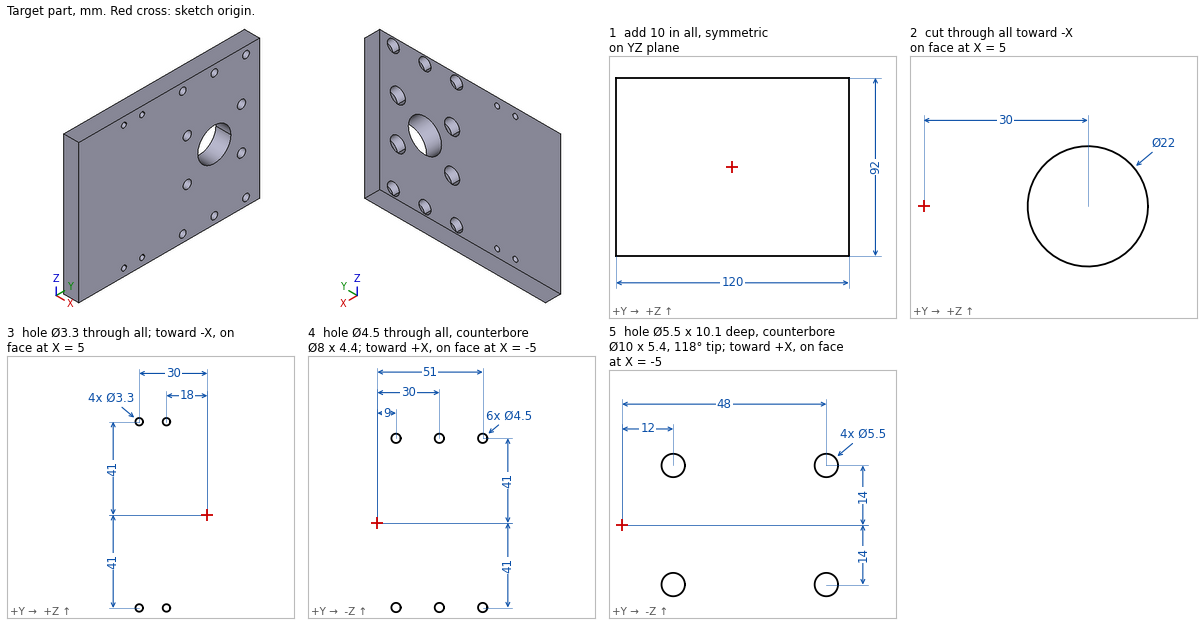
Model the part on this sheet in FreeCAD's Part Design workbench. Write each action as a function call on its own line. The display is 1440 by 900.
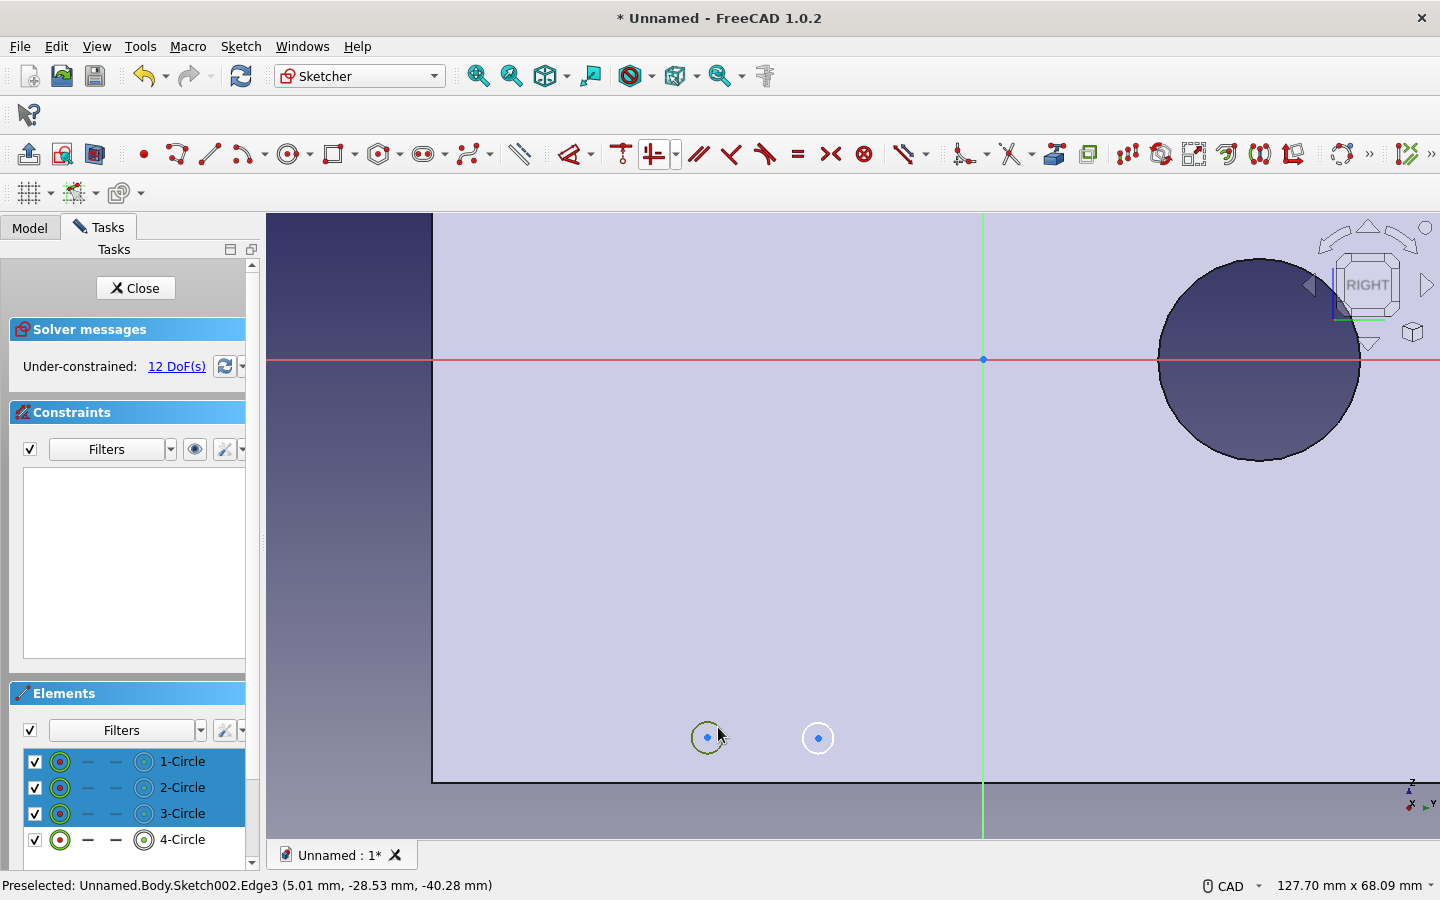
click(829, 727)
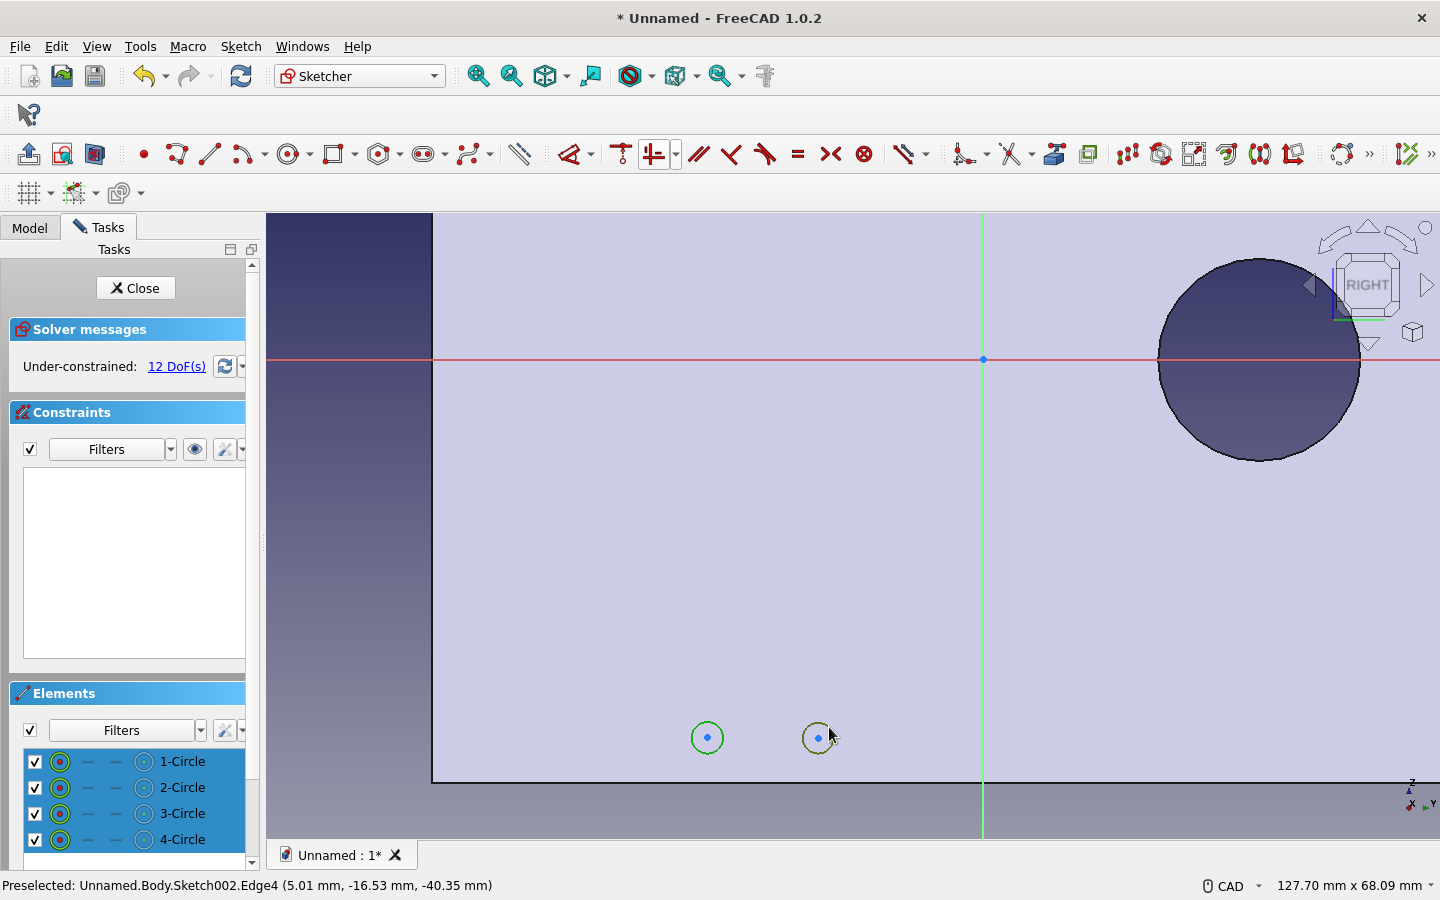
key(e)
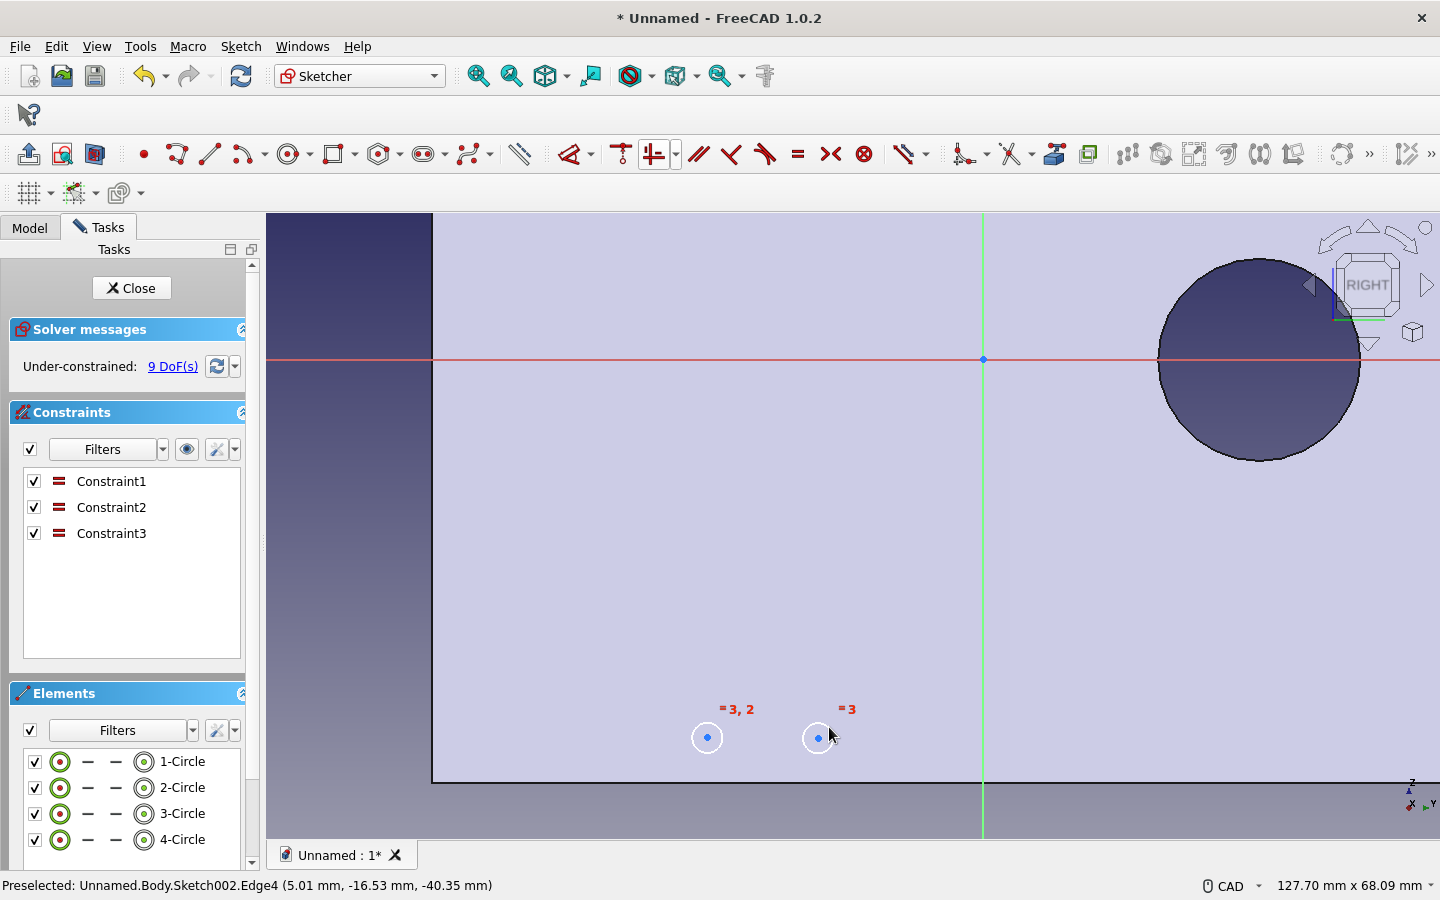
scroll(719, 728, down, 3)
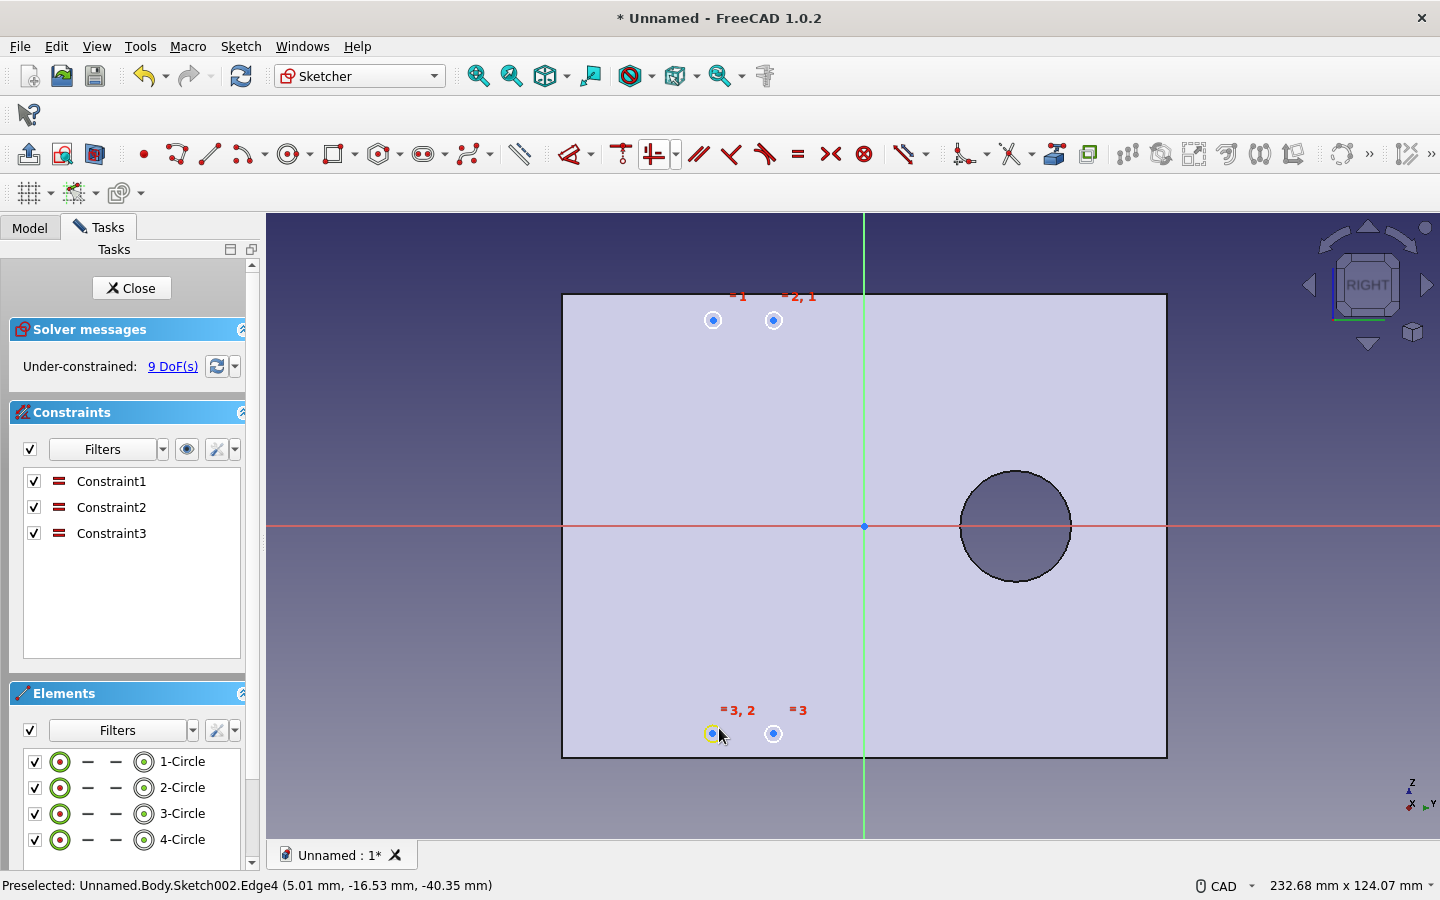
click(713, 320)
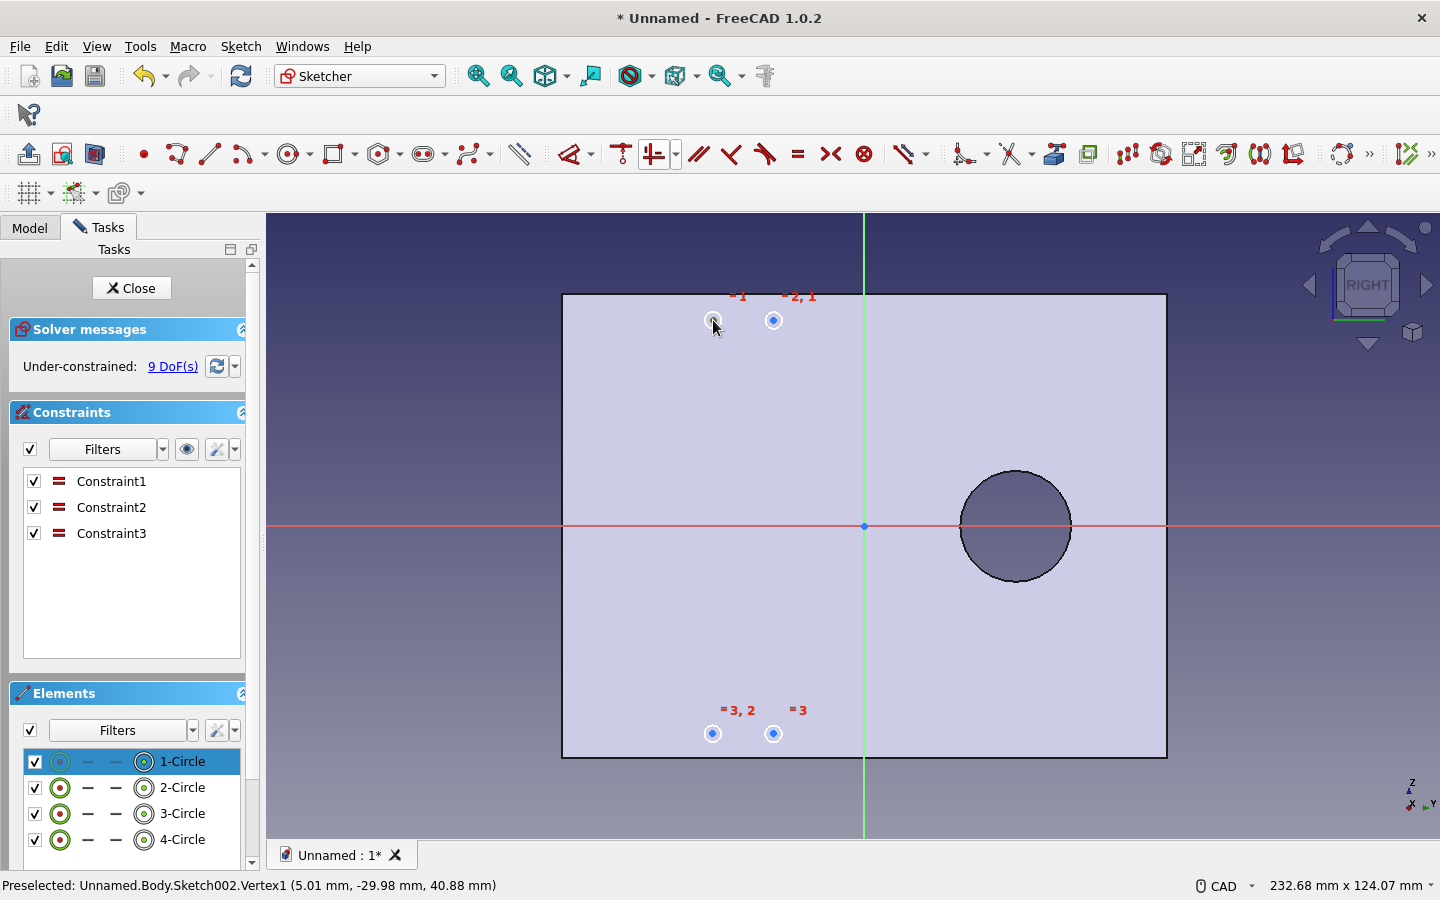
click(774, 320)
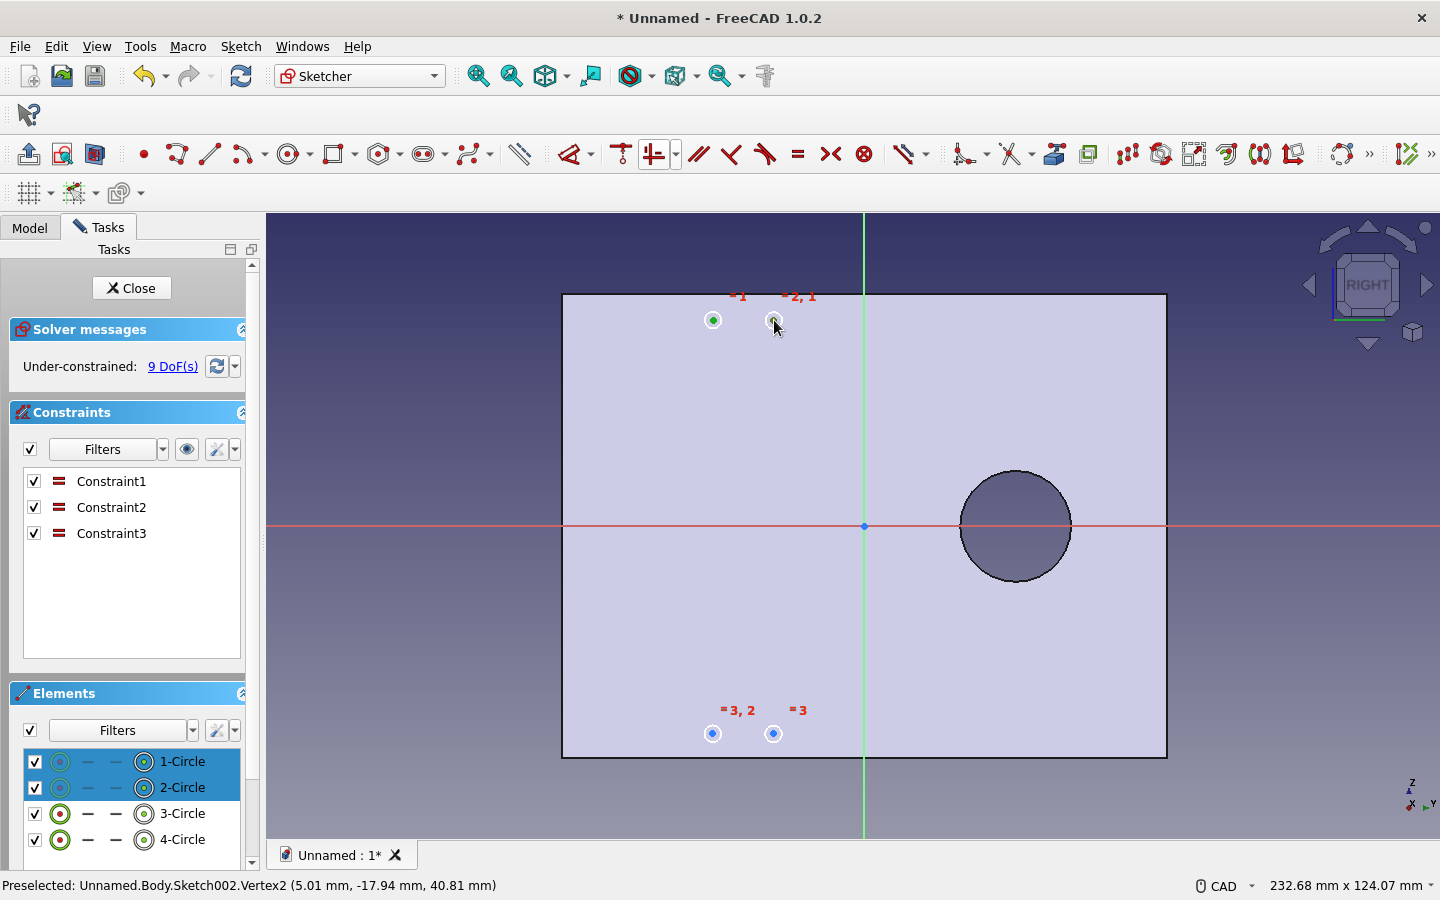
key(h)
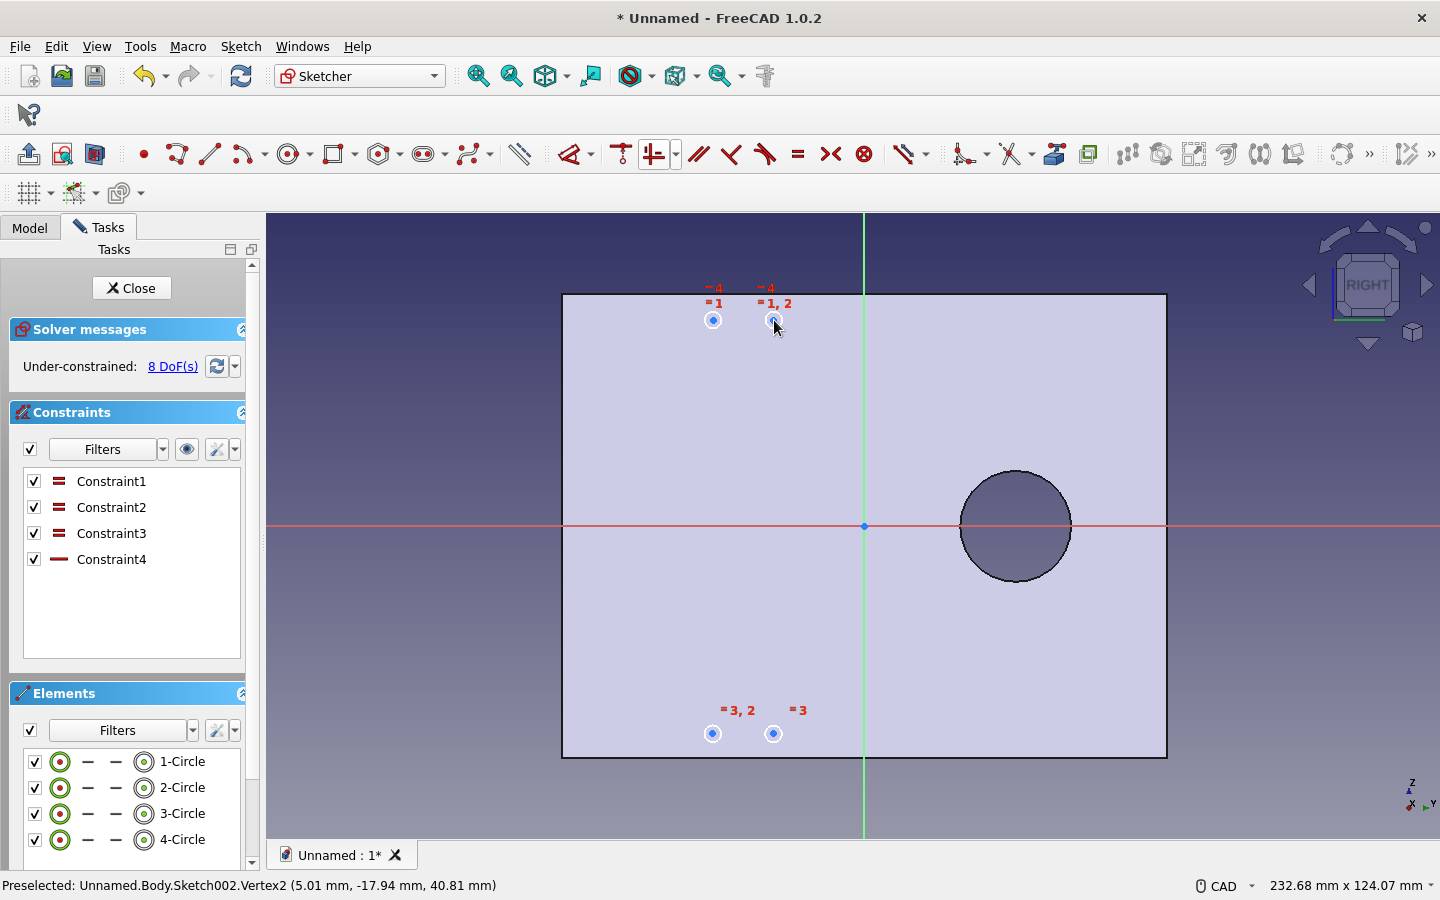
click(713, 320)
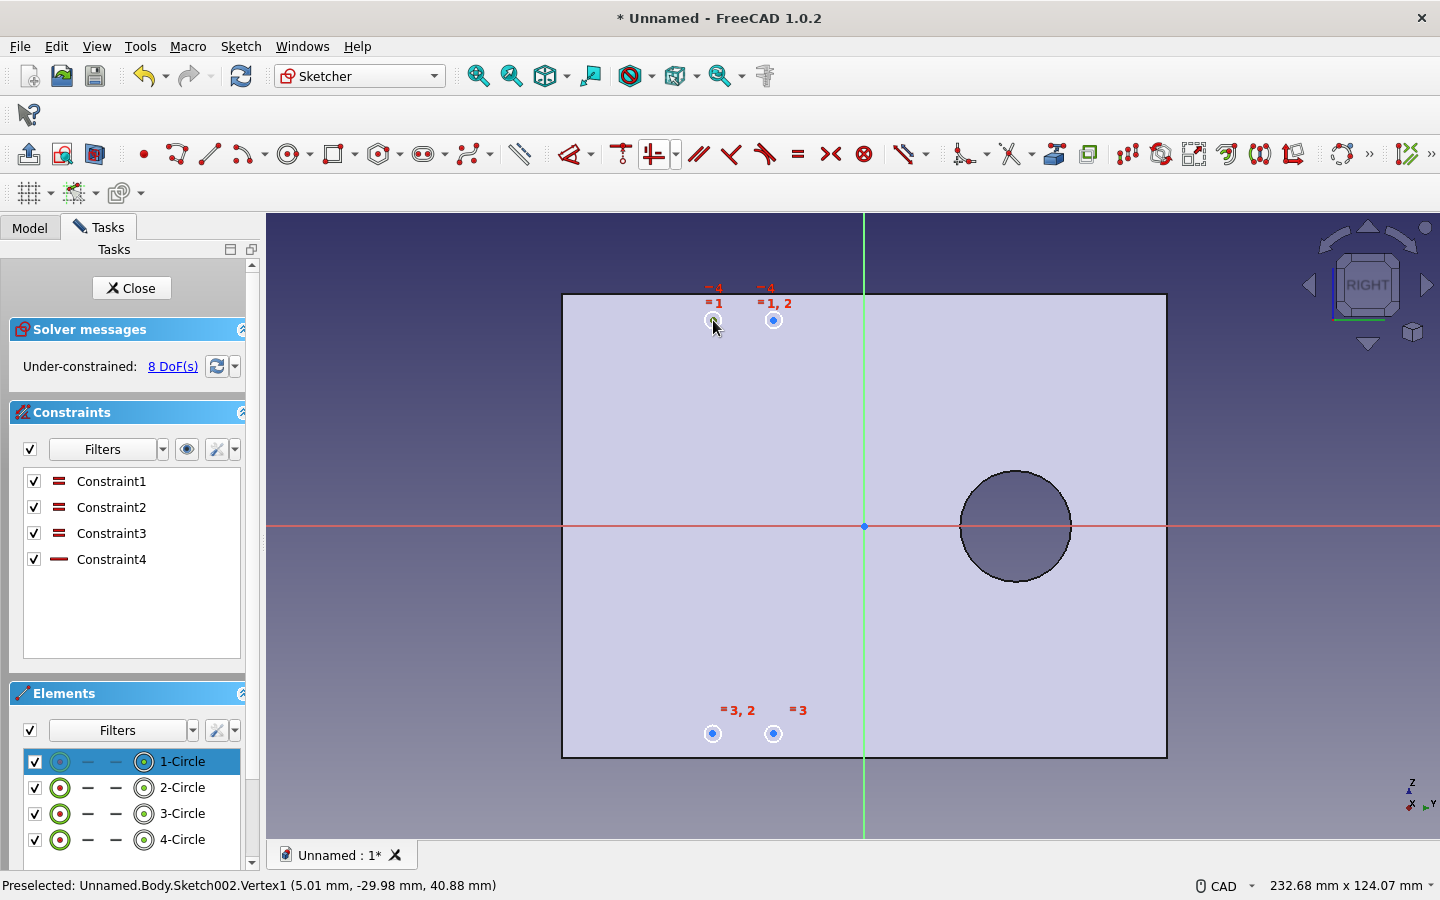
click(713, 734)